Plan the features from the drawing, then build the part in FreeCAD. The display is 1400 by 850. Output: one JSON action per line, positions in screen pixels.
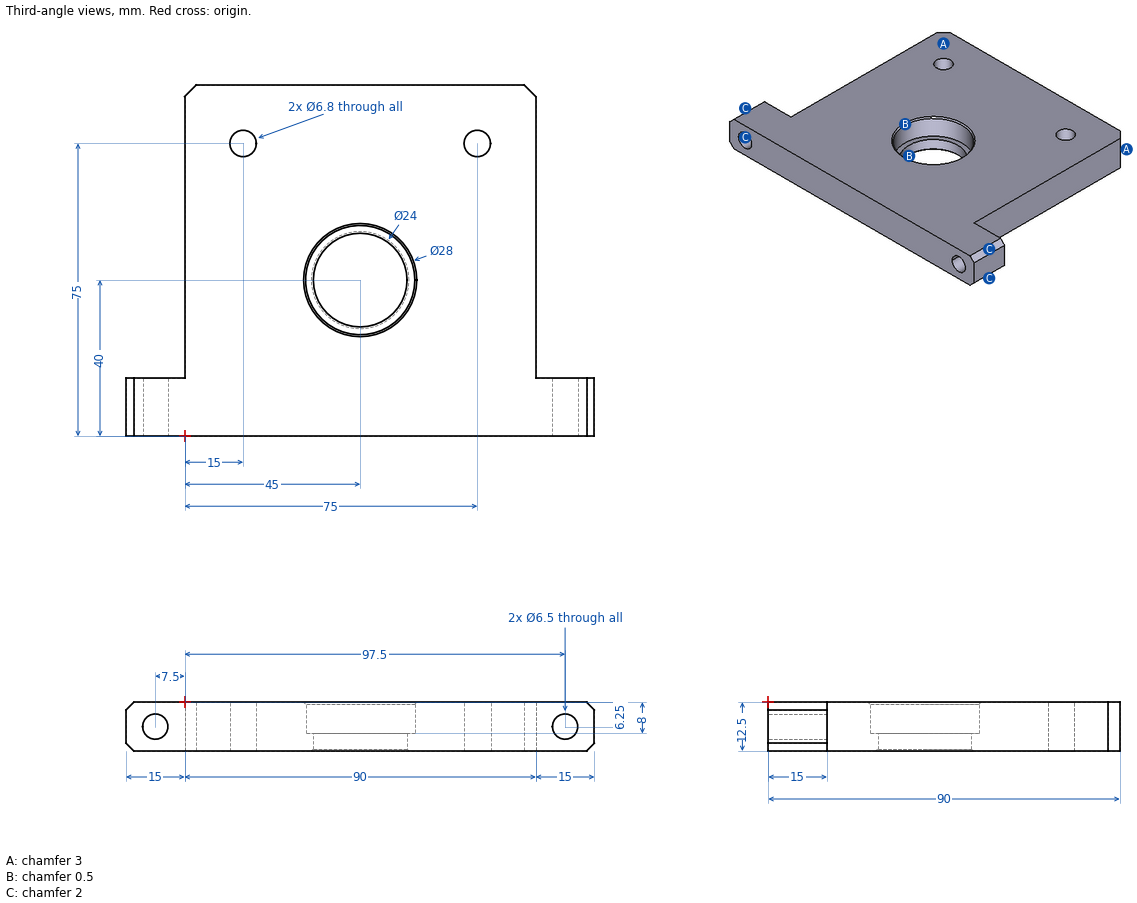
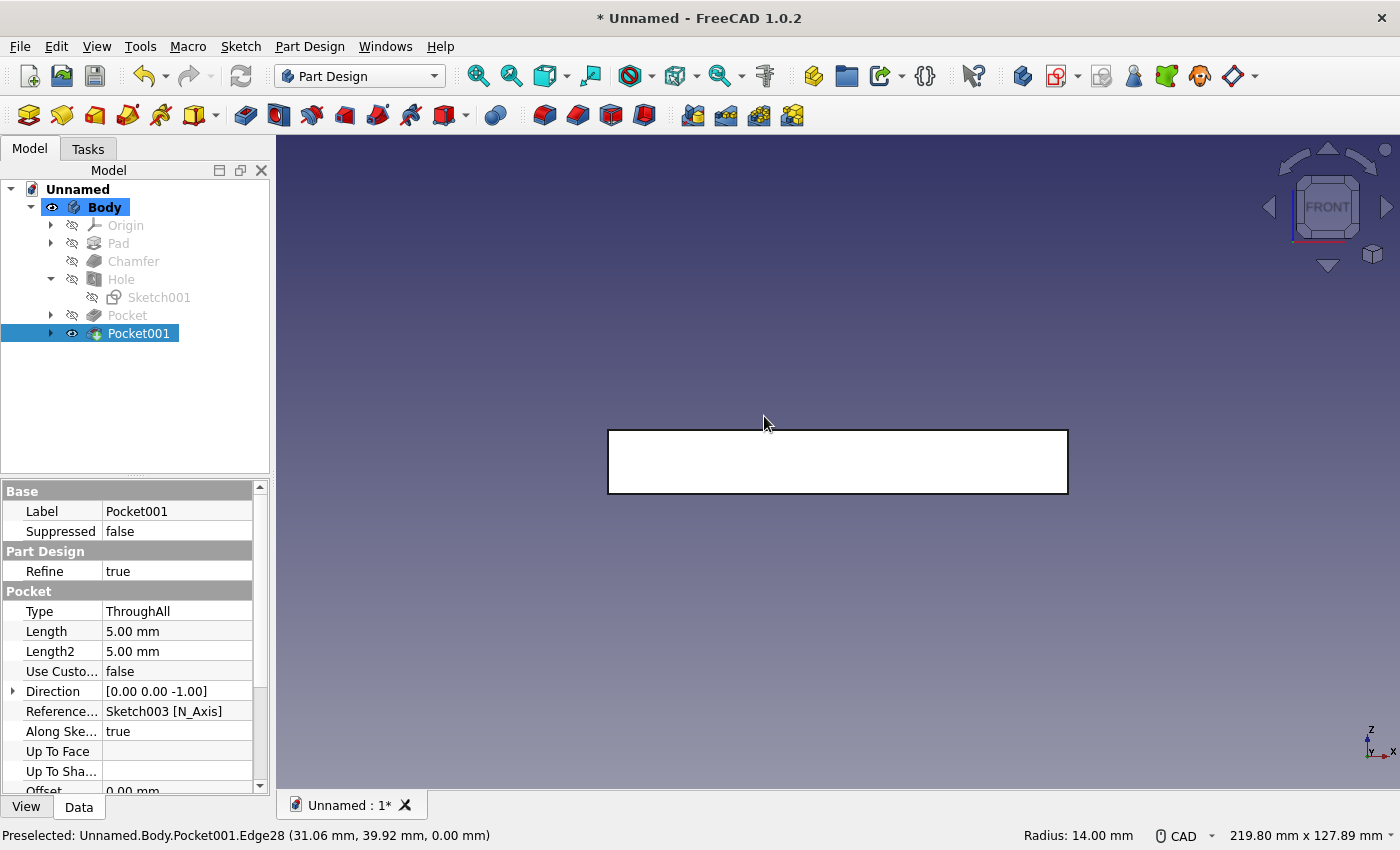
{"action": "left_click", "coordinate": [479, 76]}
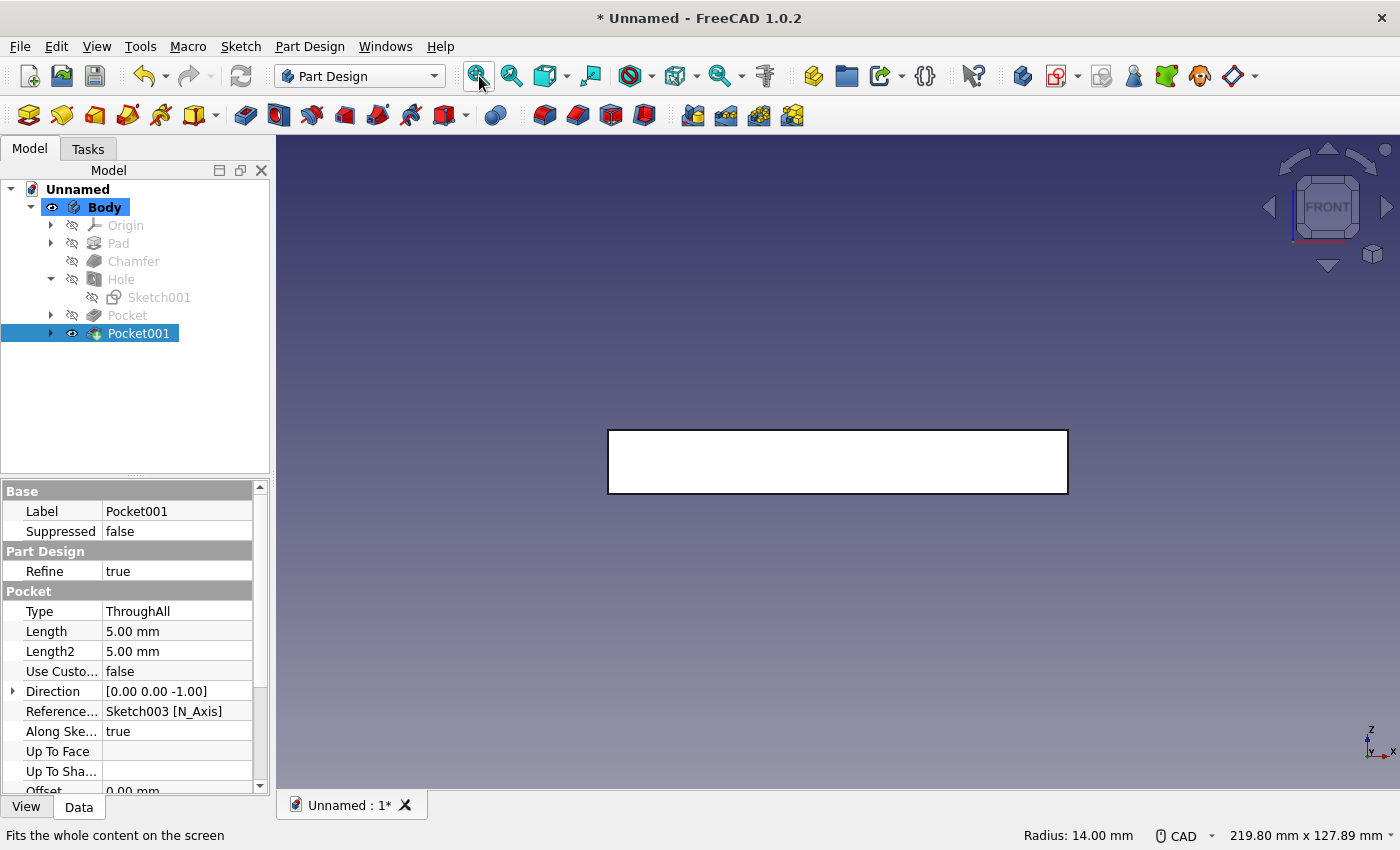
{"action": "key", "text": "3"}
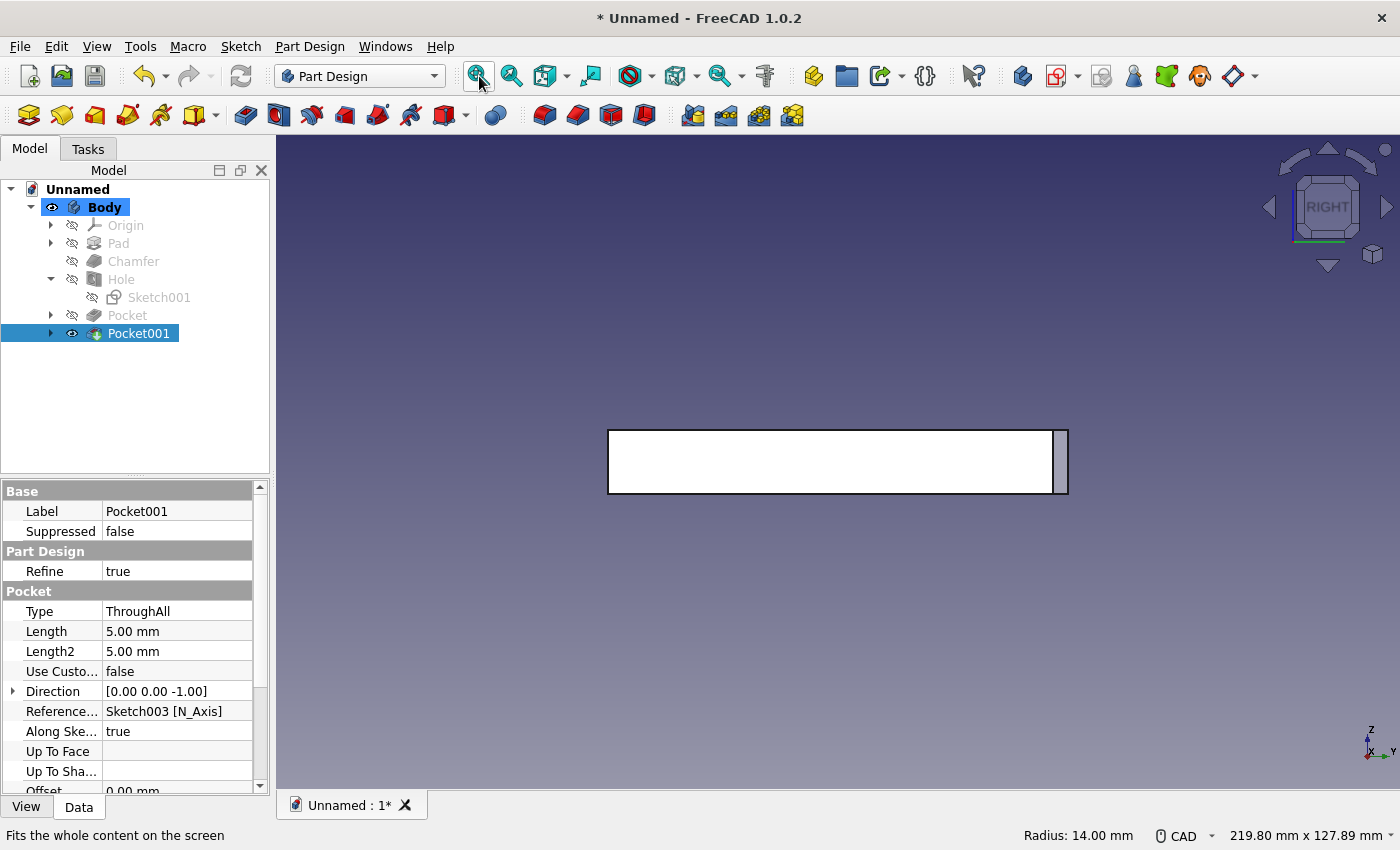
{"action": "left_click", "coordinate": [479, 76]}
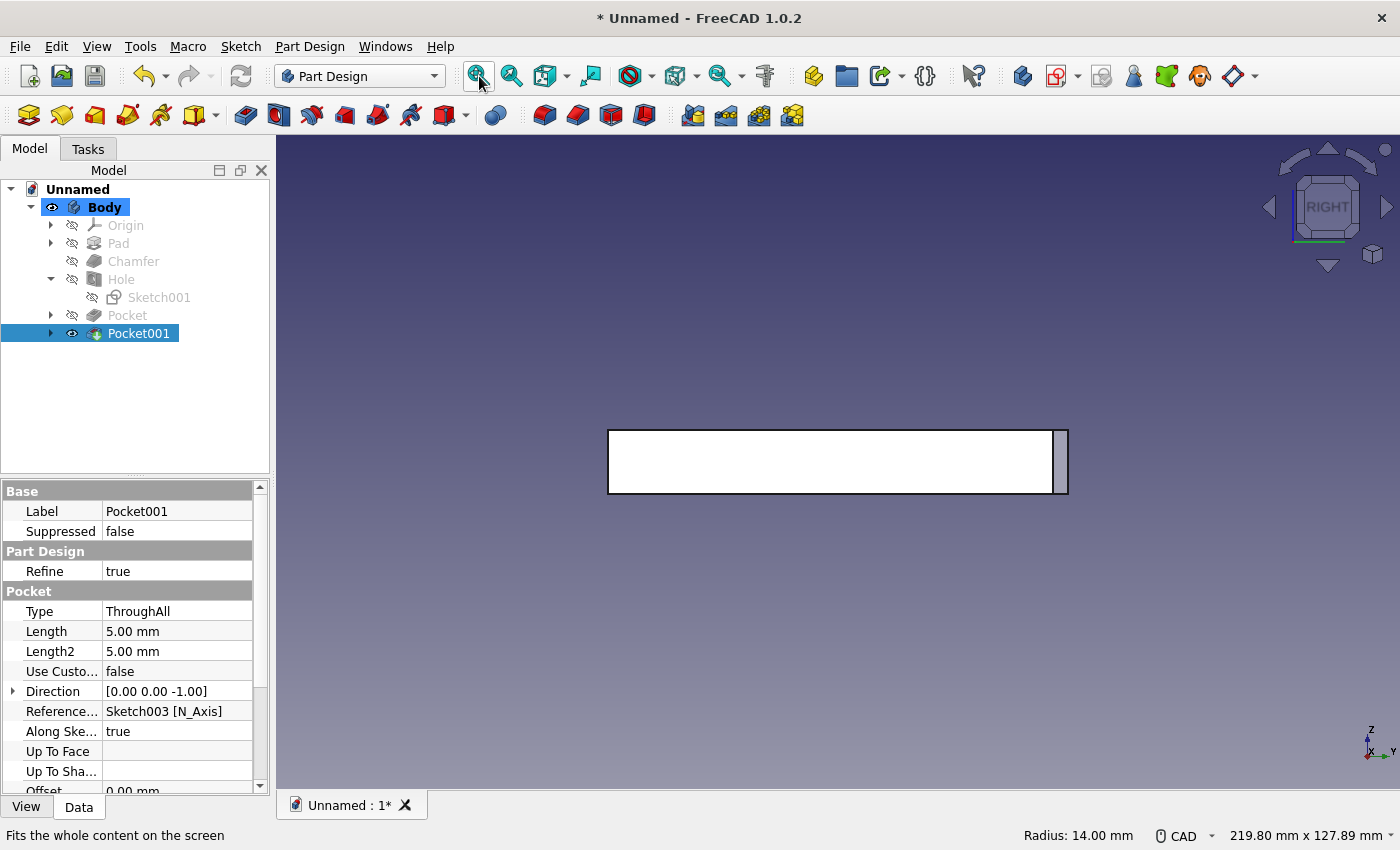
{"action": "key", "text": "5"}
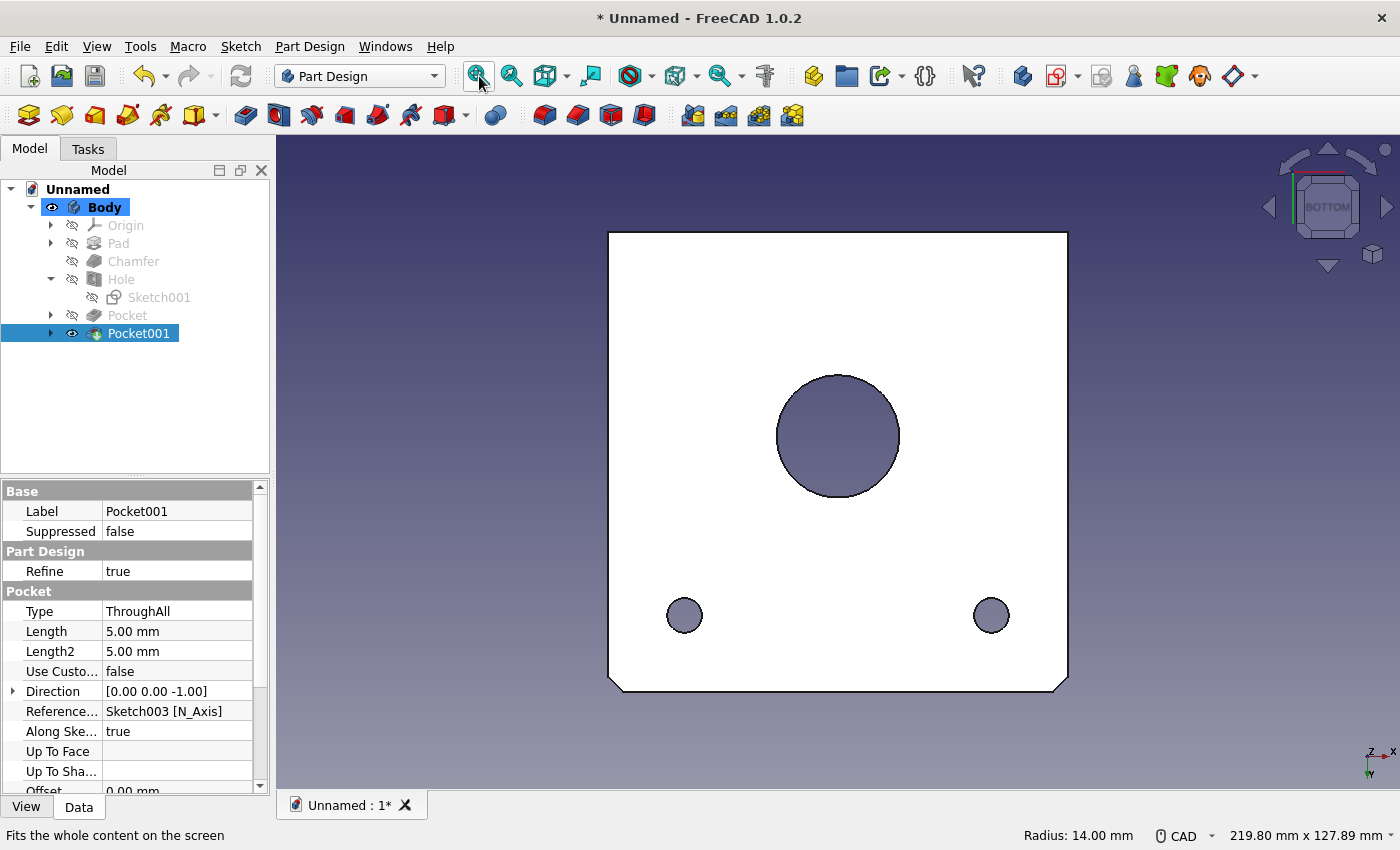
{"action": "left_click", "coordinate": [838, 497], "text": "ctrl"}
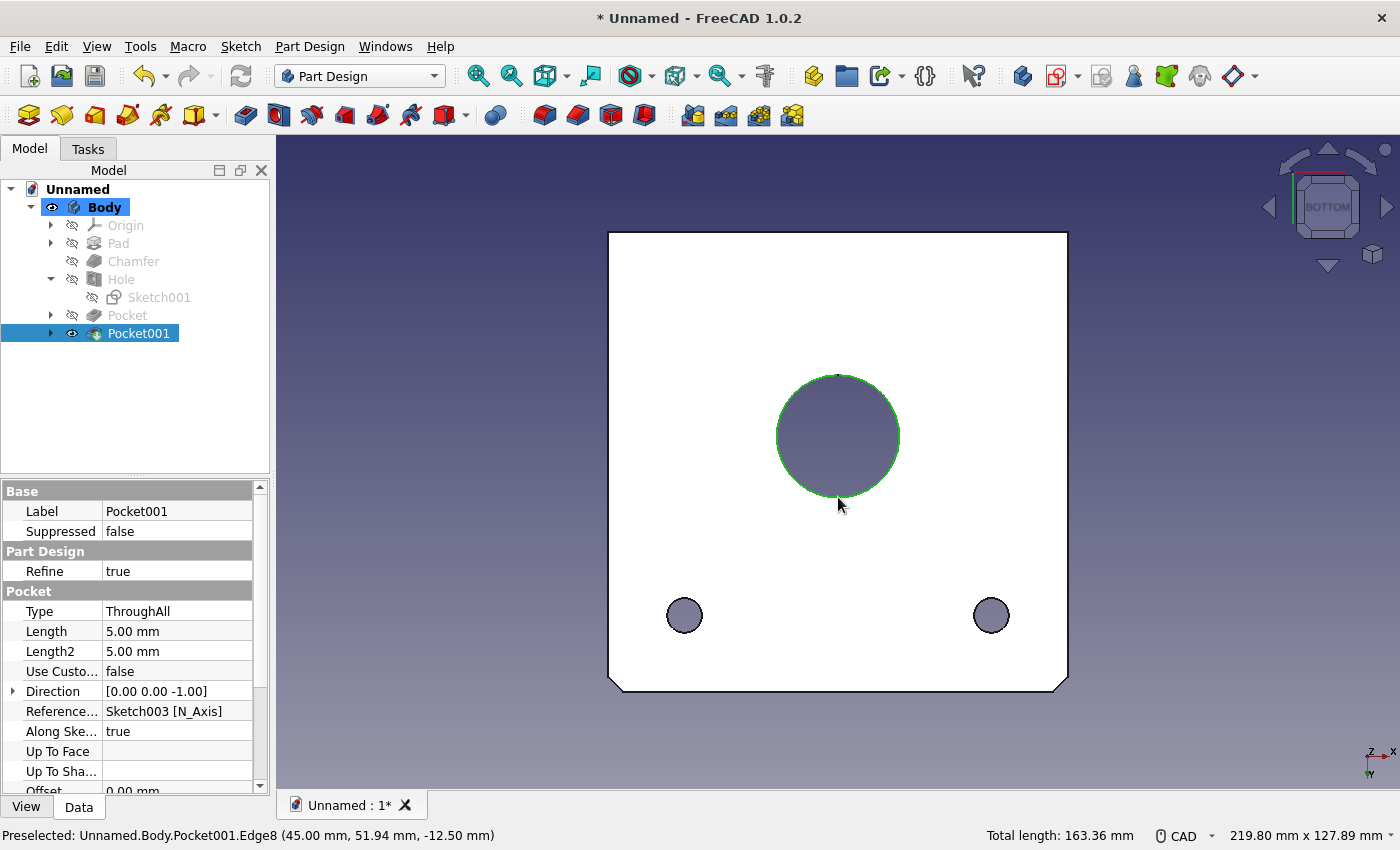
{"action": "left_click", "coordinate": [578, 116]}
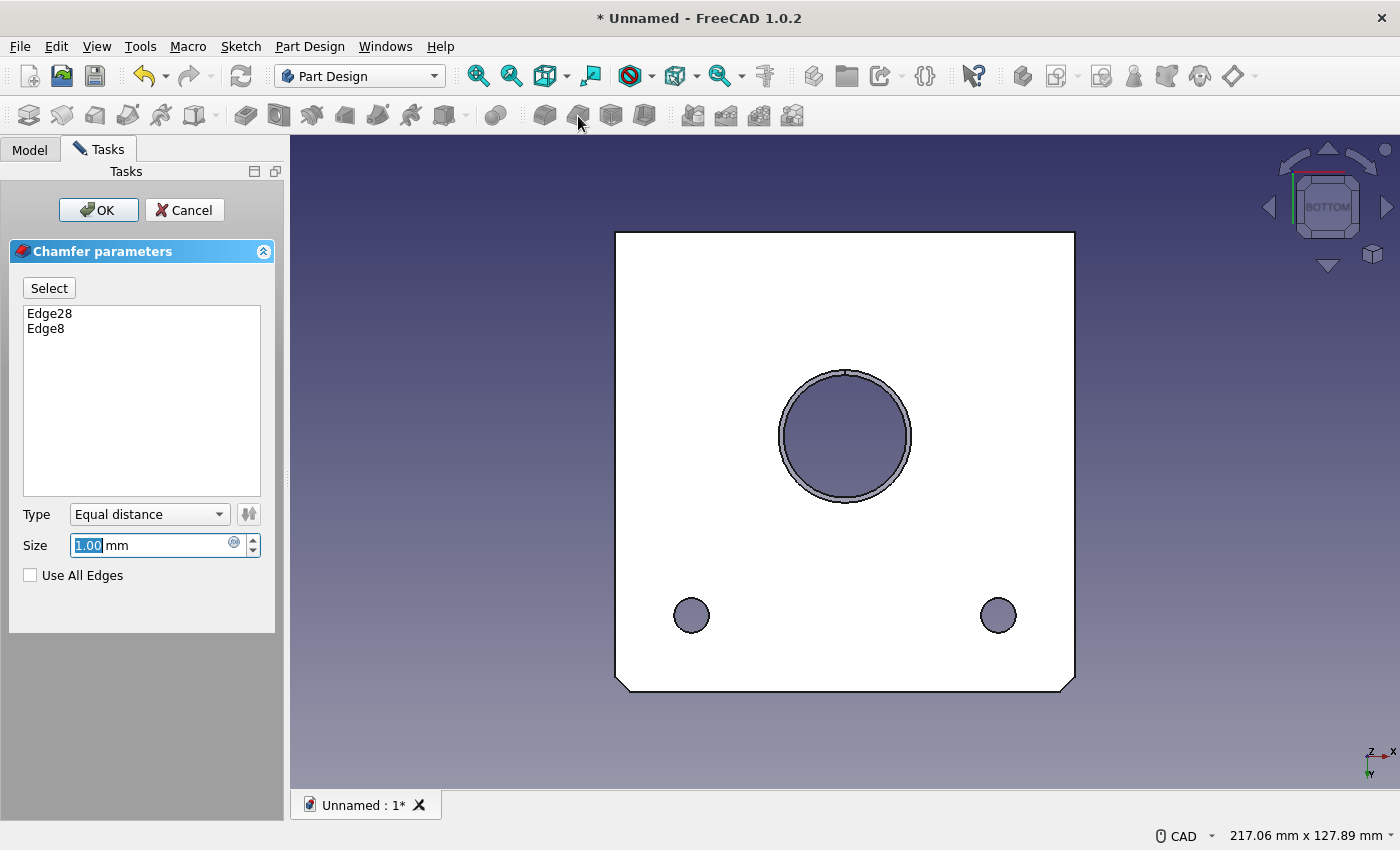
{"action": "type", "text": "0.5"}
{"action": "key", "text": "Tab"}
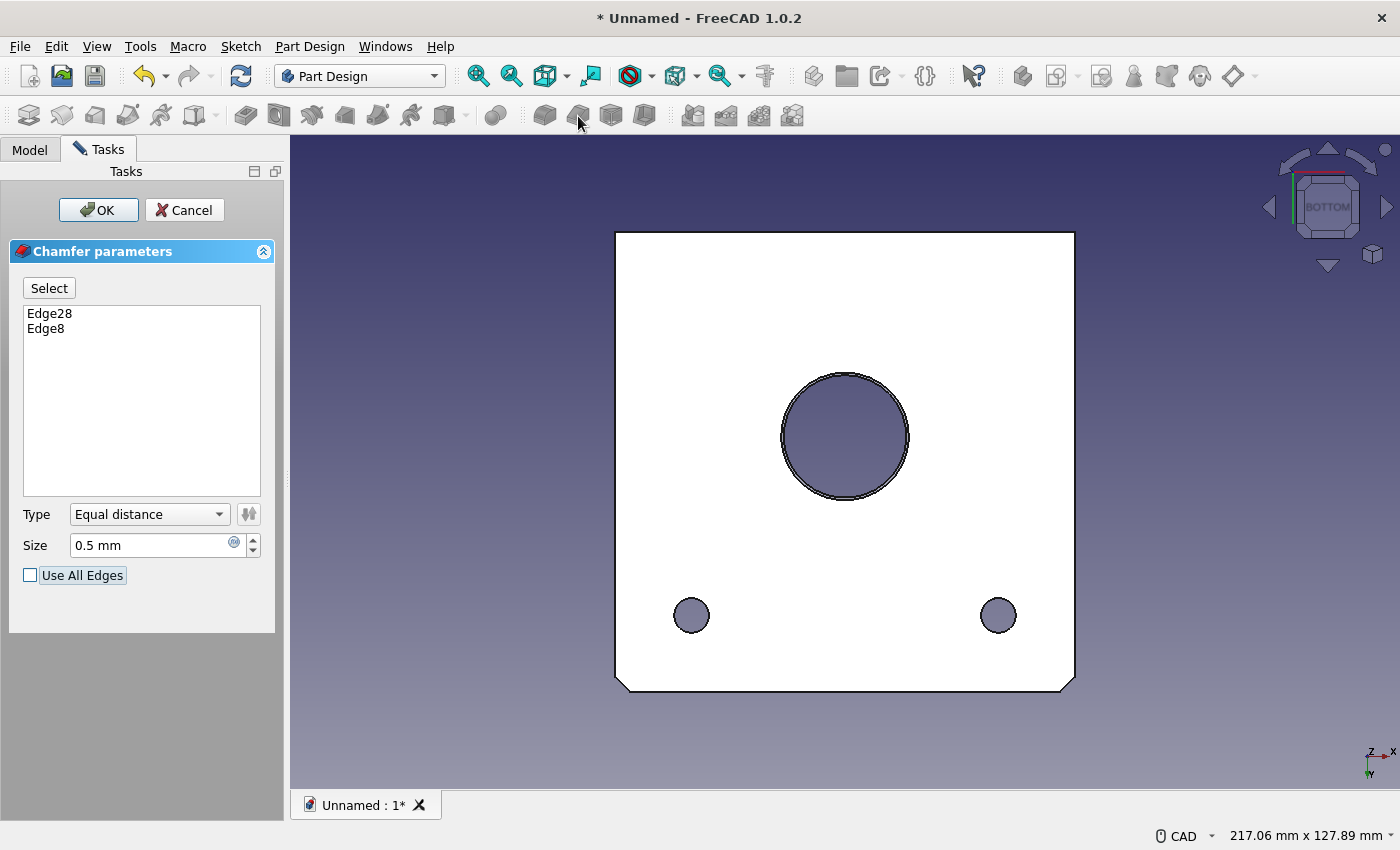
{"action": "left_click", "coordinate": [99, 210]}